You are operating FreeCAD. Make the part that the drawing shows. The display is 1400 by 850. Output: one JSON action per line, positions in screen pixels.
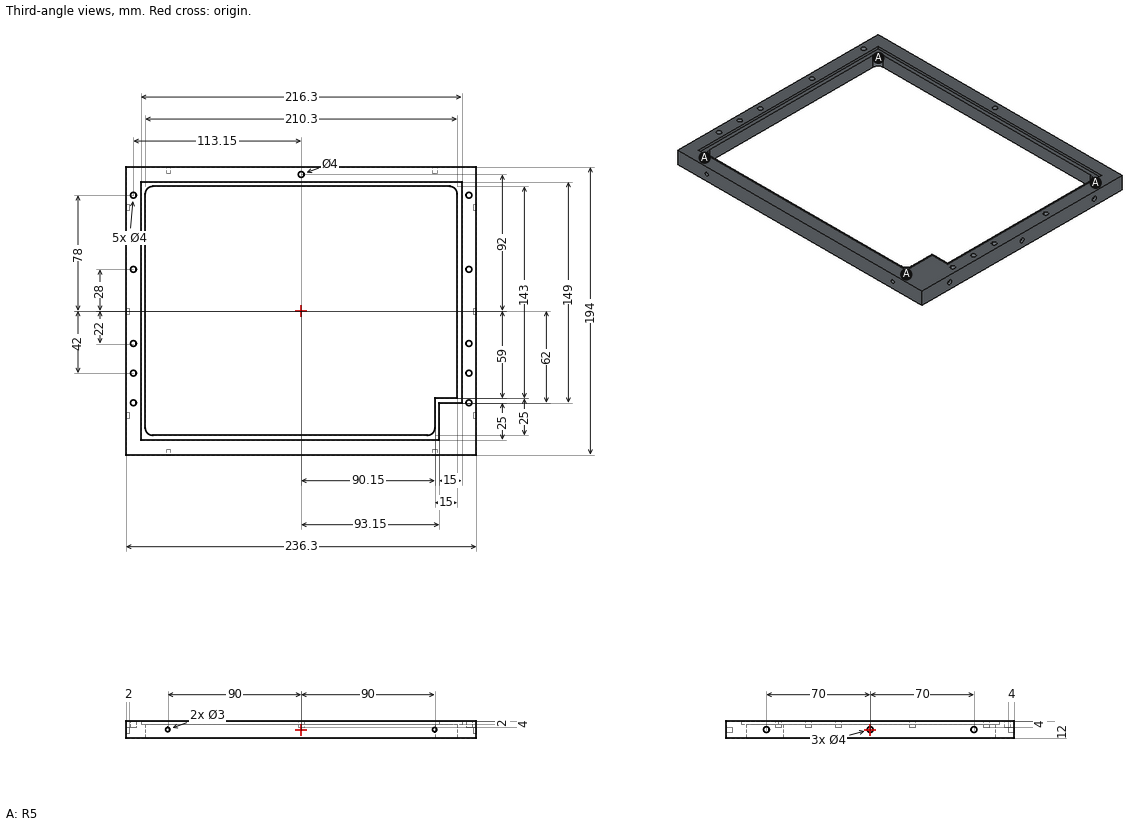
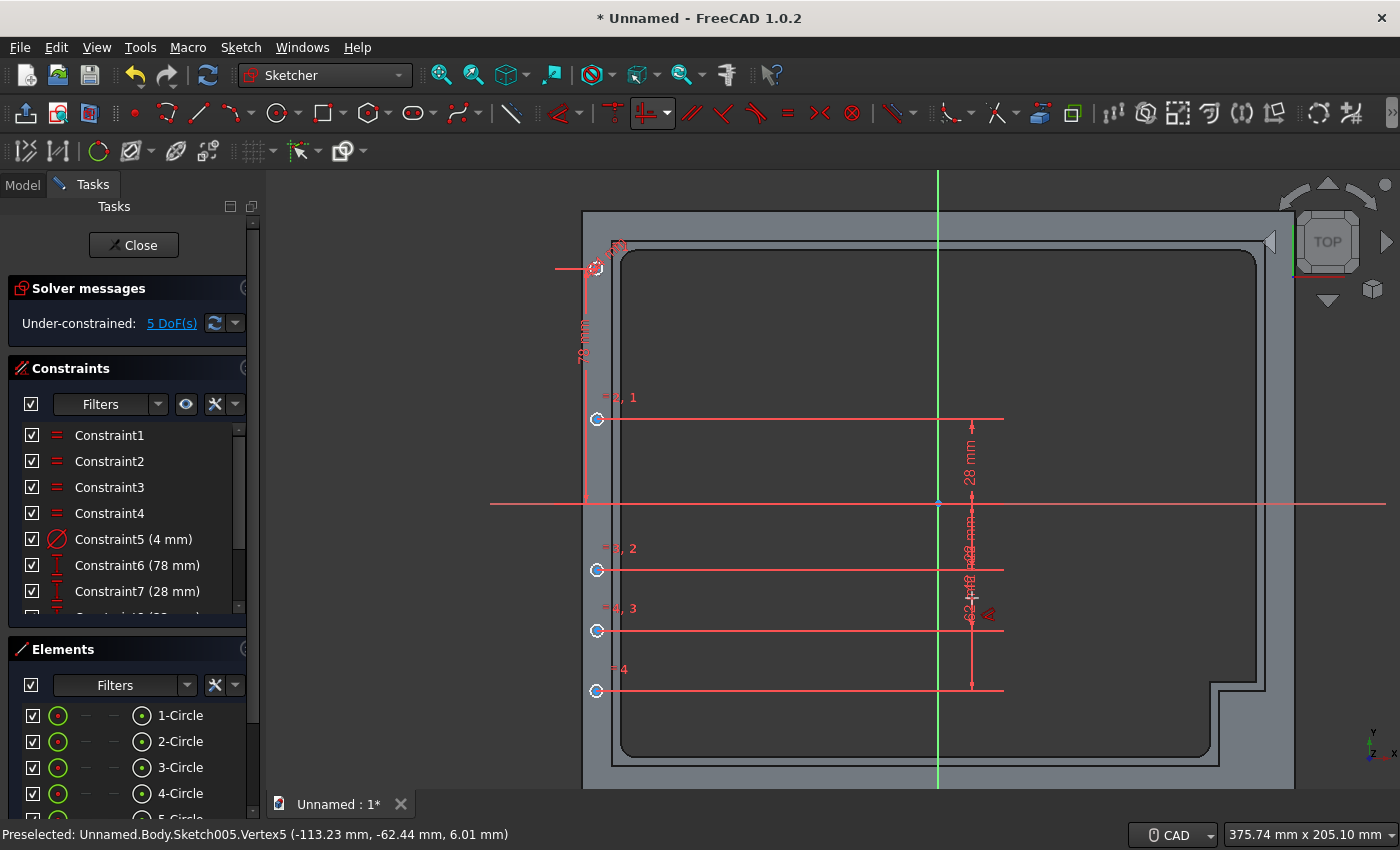
{"action": "left_click", "coordinate": [596, 269]}
{"action": "left_click", "coordinate": [767, 235]}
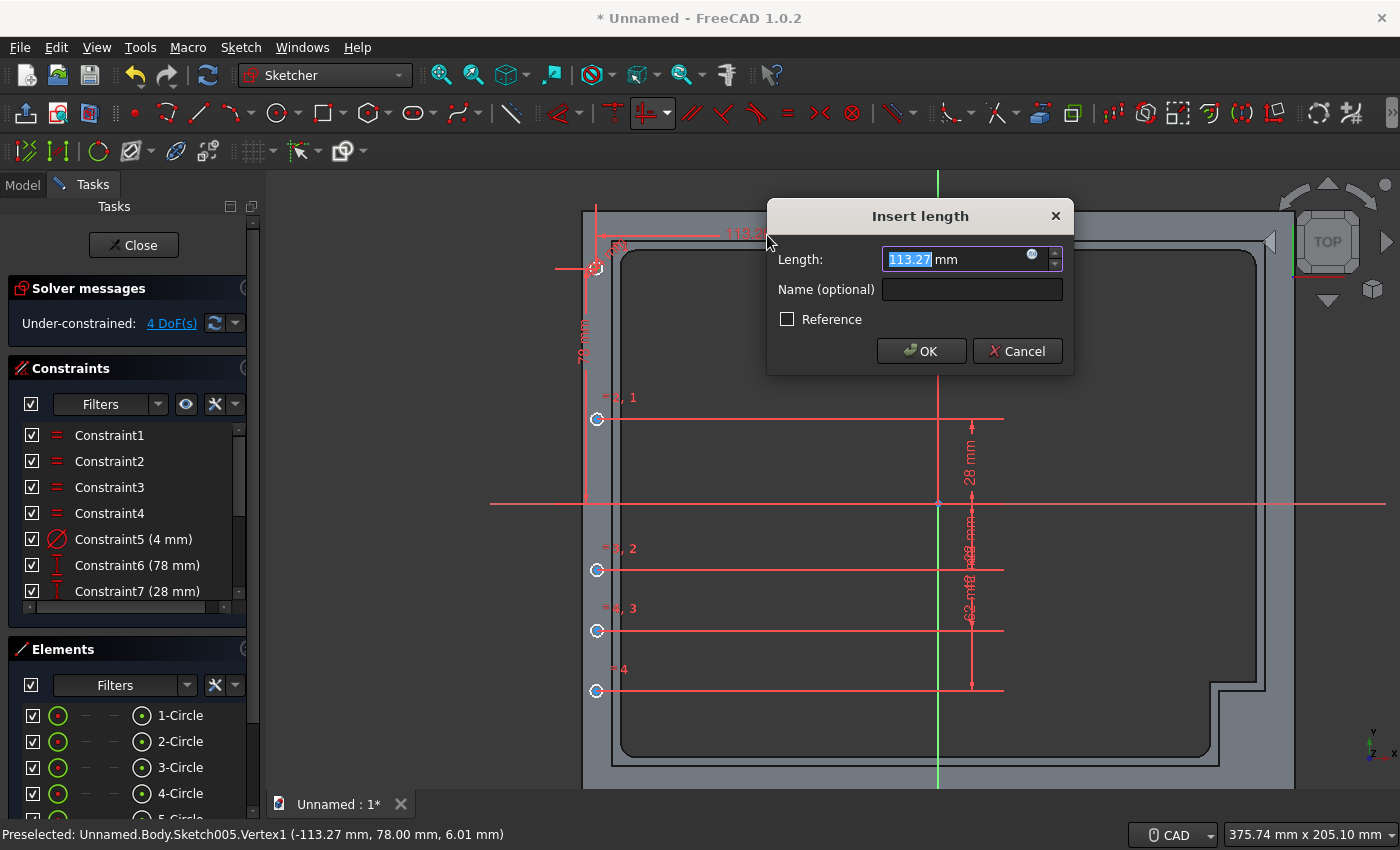
{"action": "type", "text": "113.15"}
{"action": "key", "text": "Return"}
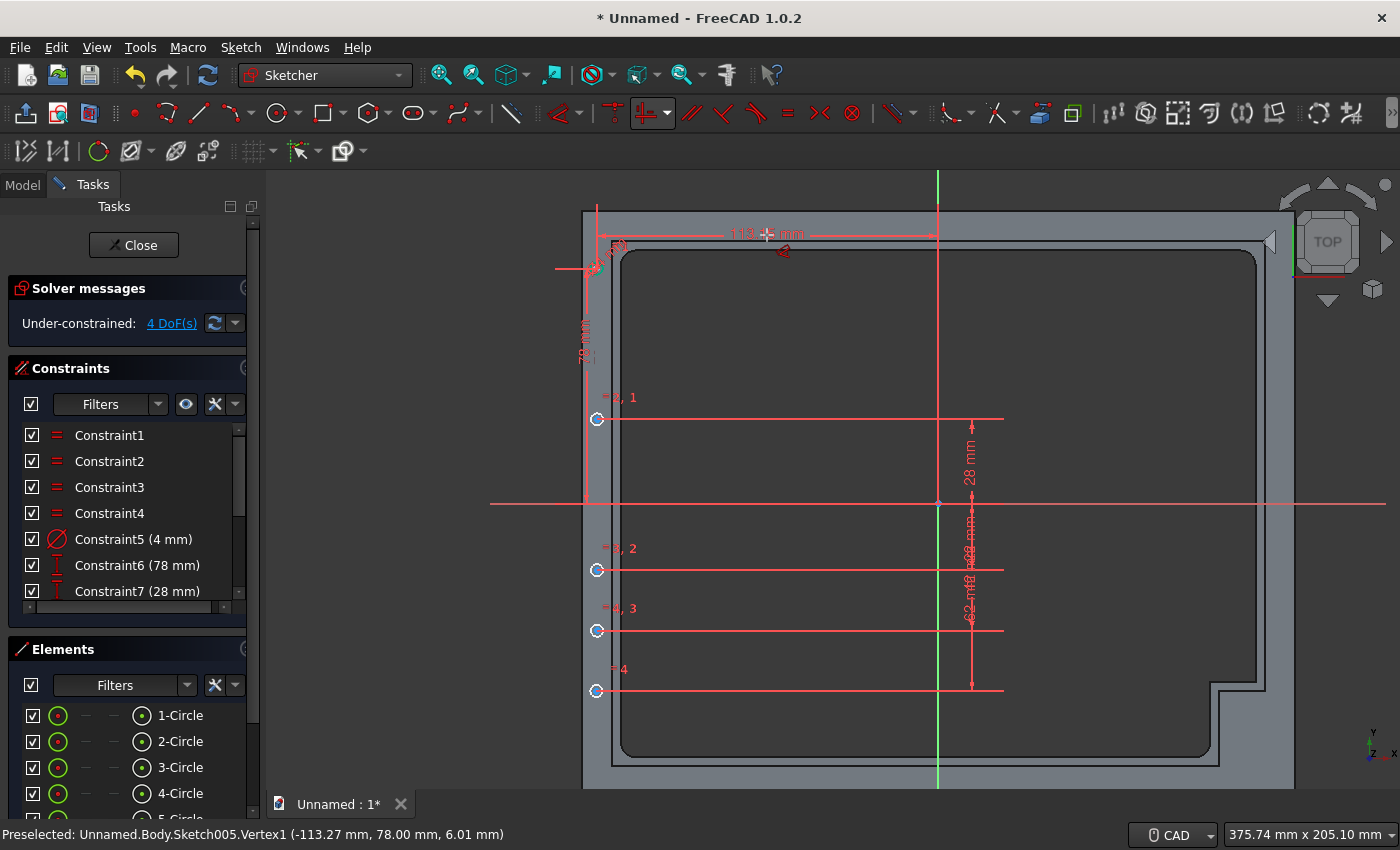
{"action": "left_click", "coordinate": [597, 419]}
{"action": "left_click", "coordinate": [768, 385]}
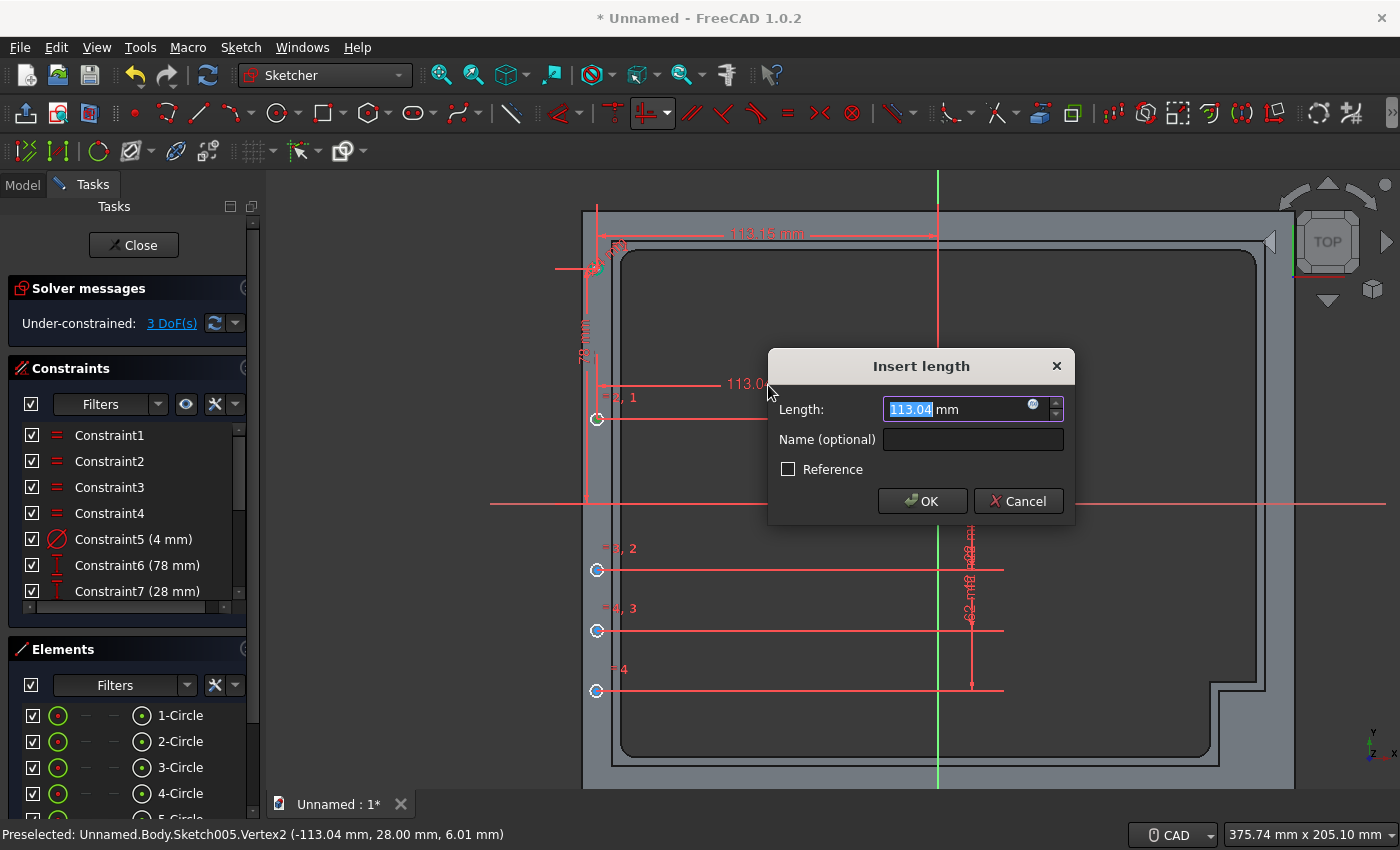
{"action": "type", "text": "113.15"}
{"action": "key", "text": "Return"}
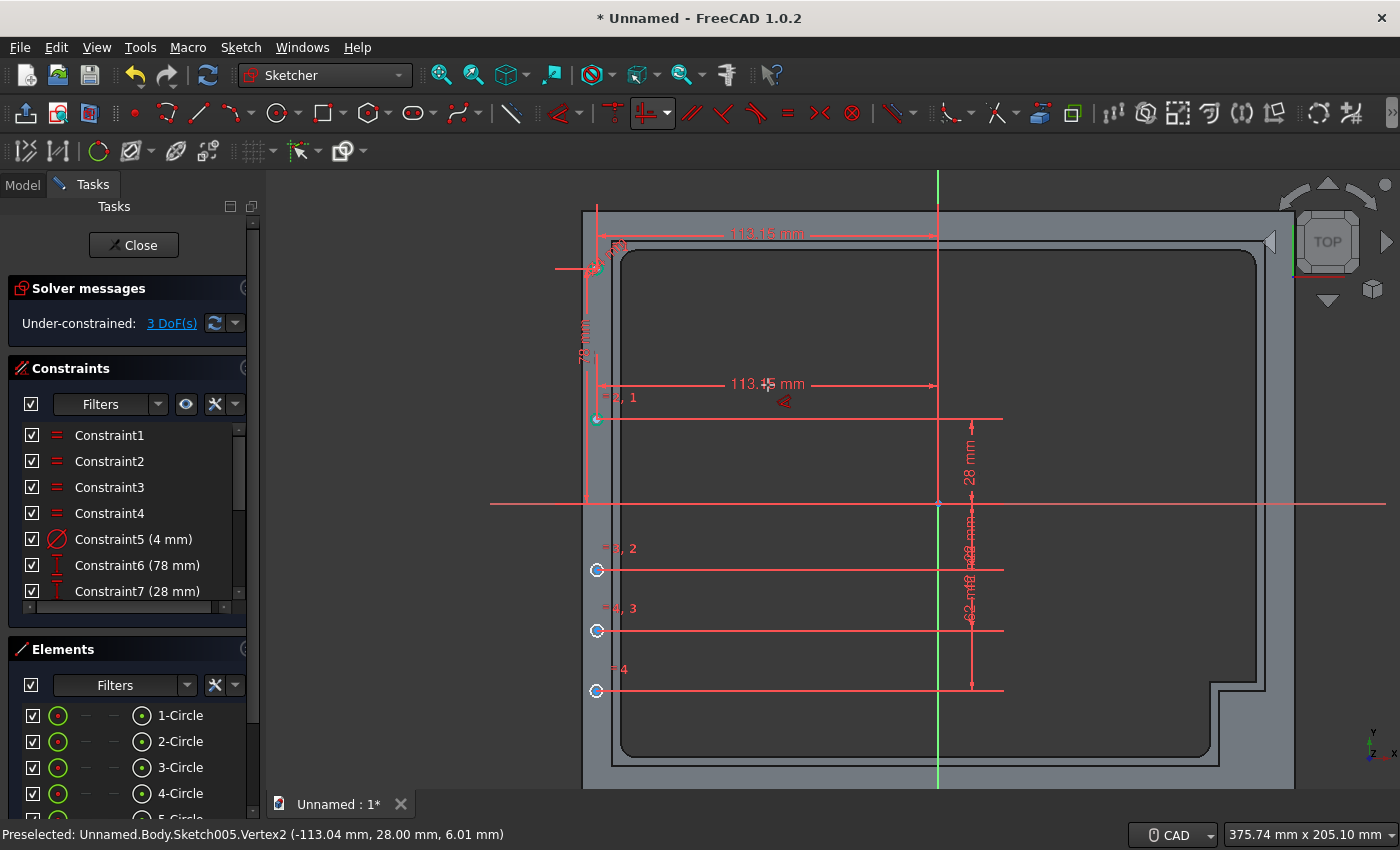
{"action": "left_click", "coordinate": [597, 570]}
{"action": "left_click", "coordinate": [768, 604]}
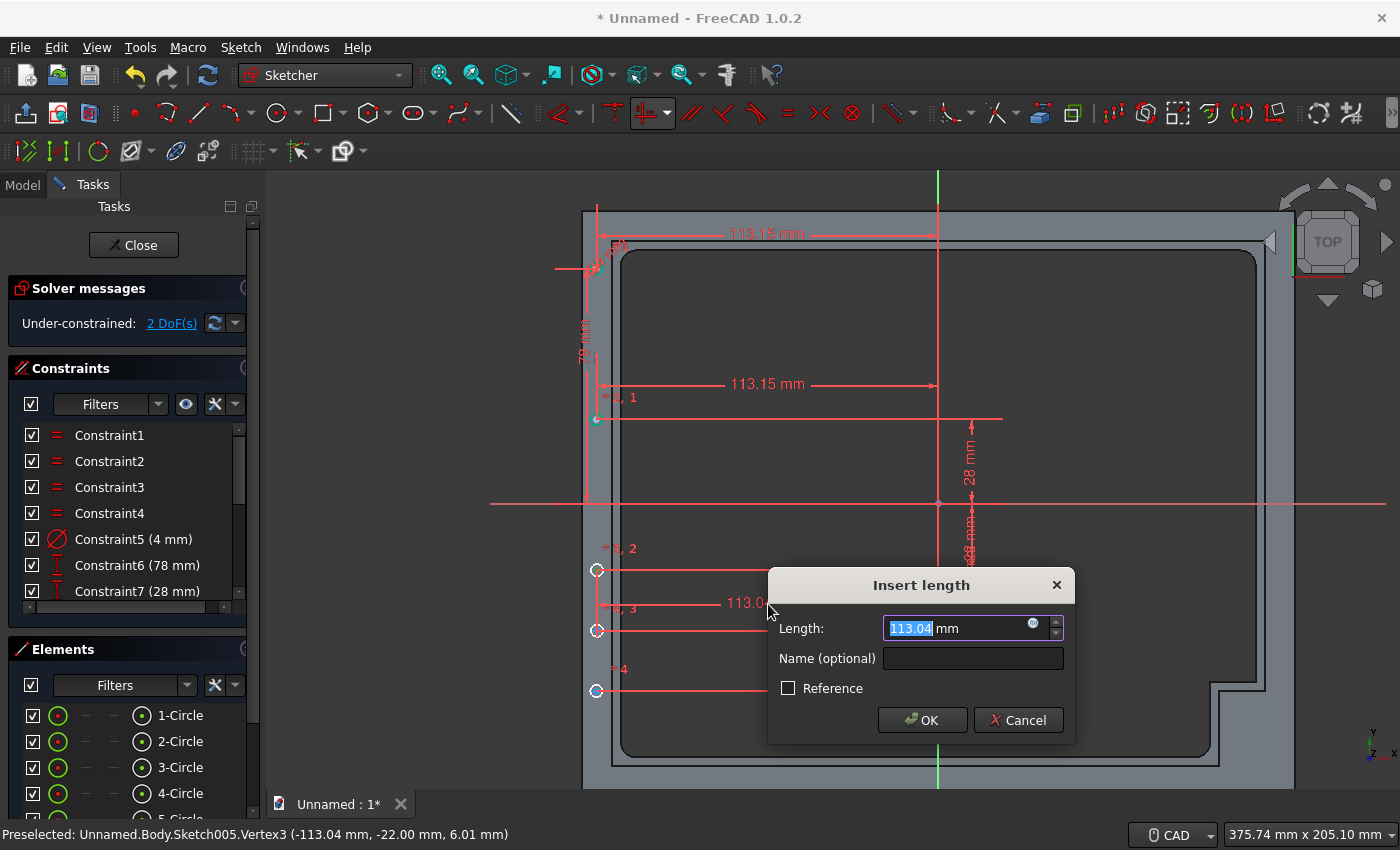
{"action": "type", "text": "113.15"}
{"action": "key", "text": "Return"}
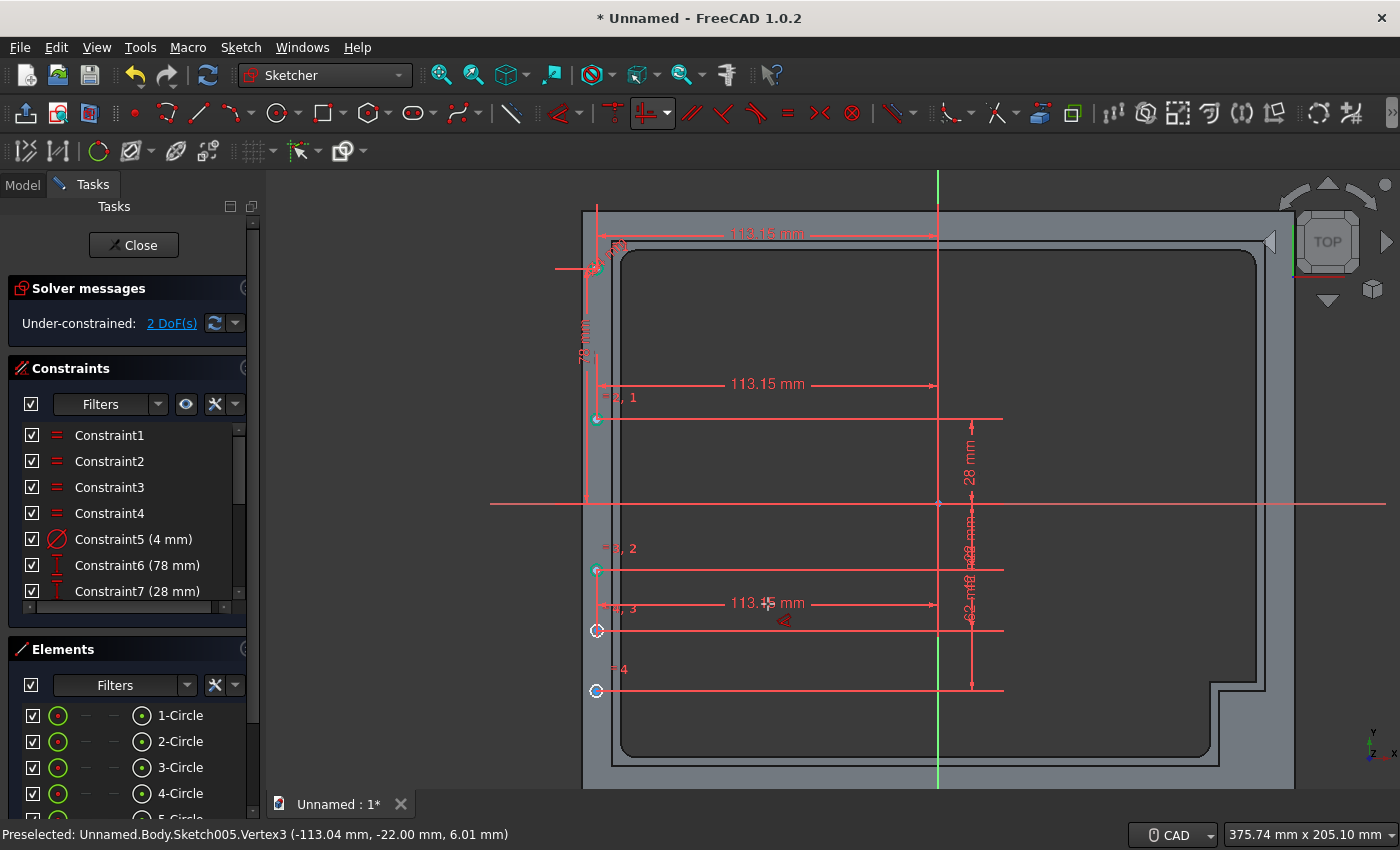
{"action": "left_click", "coordinate": [597, 631]}
{"action": "left_click", "coordinate": [768, 665]}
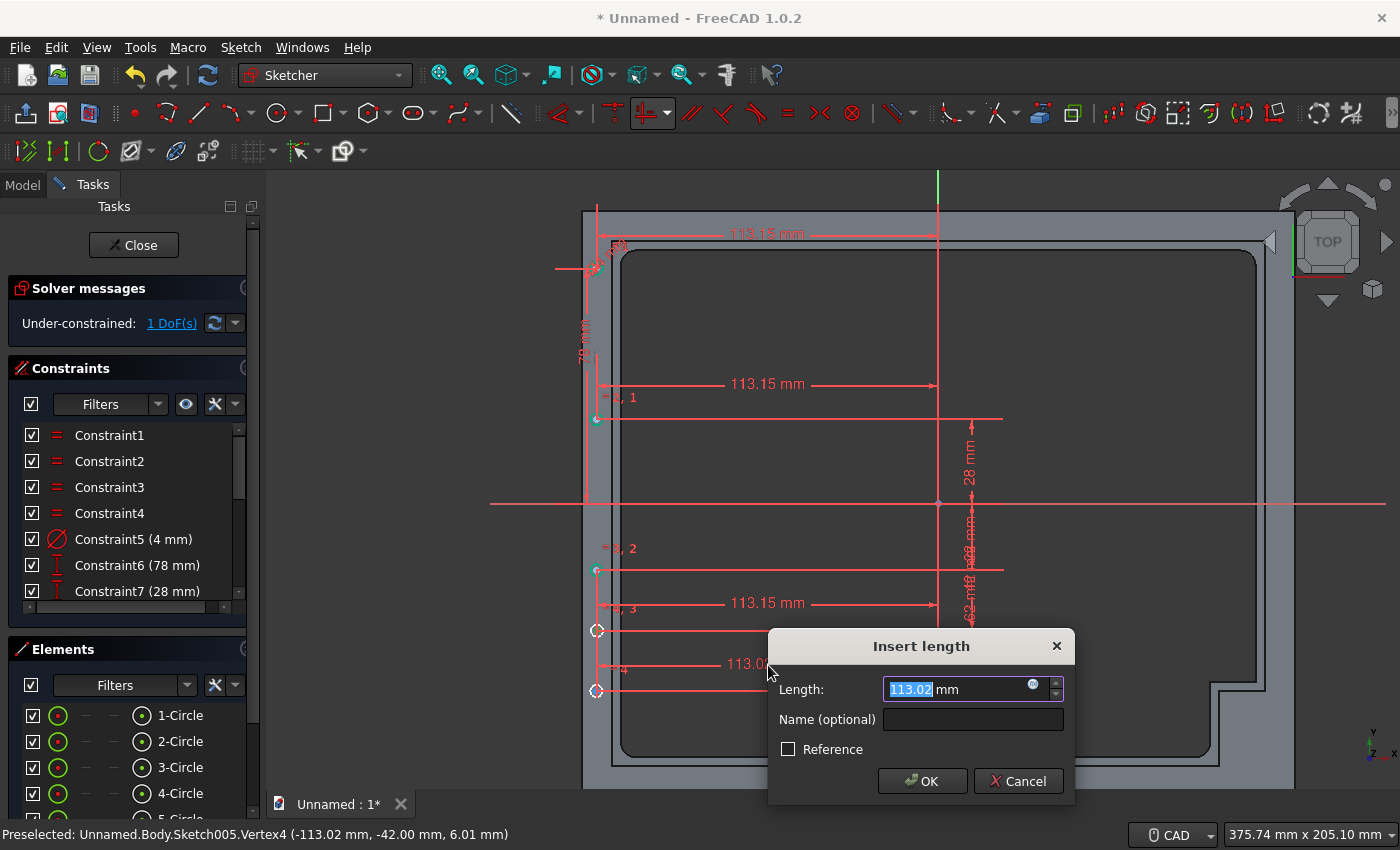
{"action": "type", "text": "113.15"}
{"action": "key", "text": "Return"}